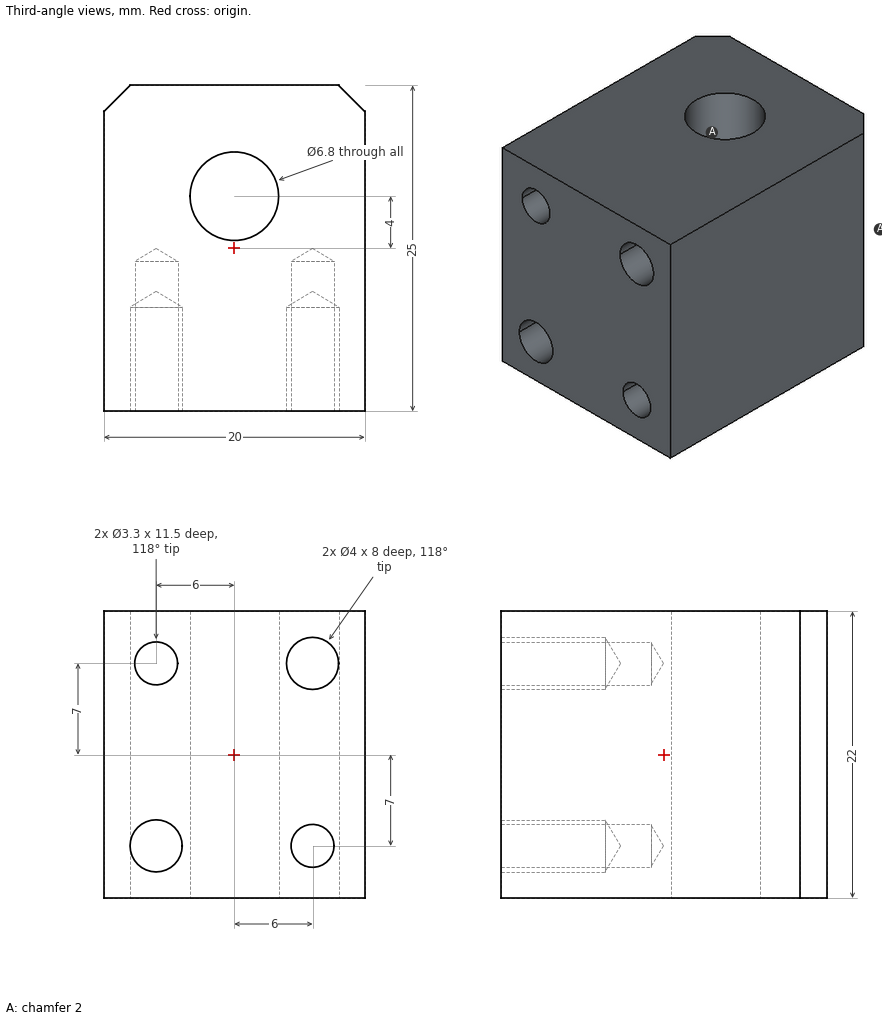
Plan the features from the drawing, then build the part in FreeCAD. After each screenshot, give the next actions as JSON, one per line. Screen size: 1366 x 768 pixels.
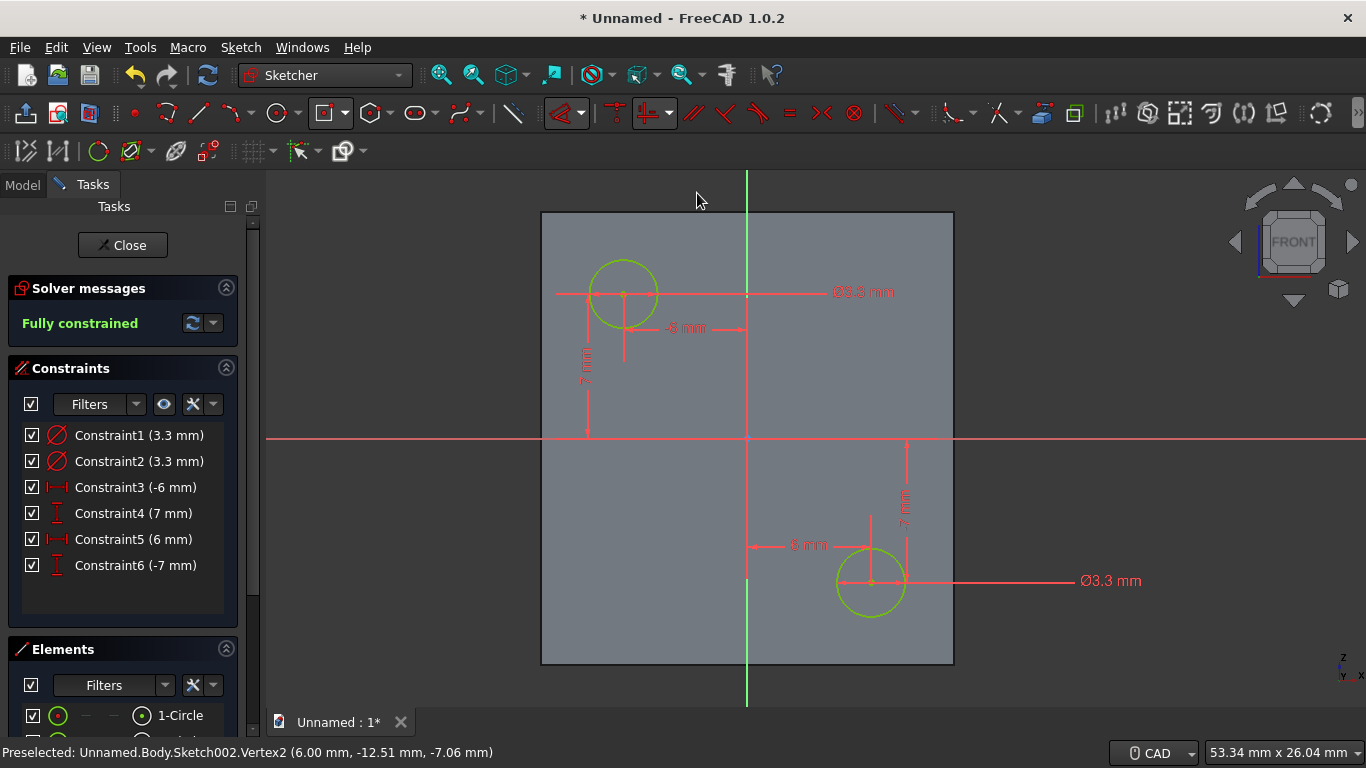
{"action": "left_click", "coordinate": [123, 245]}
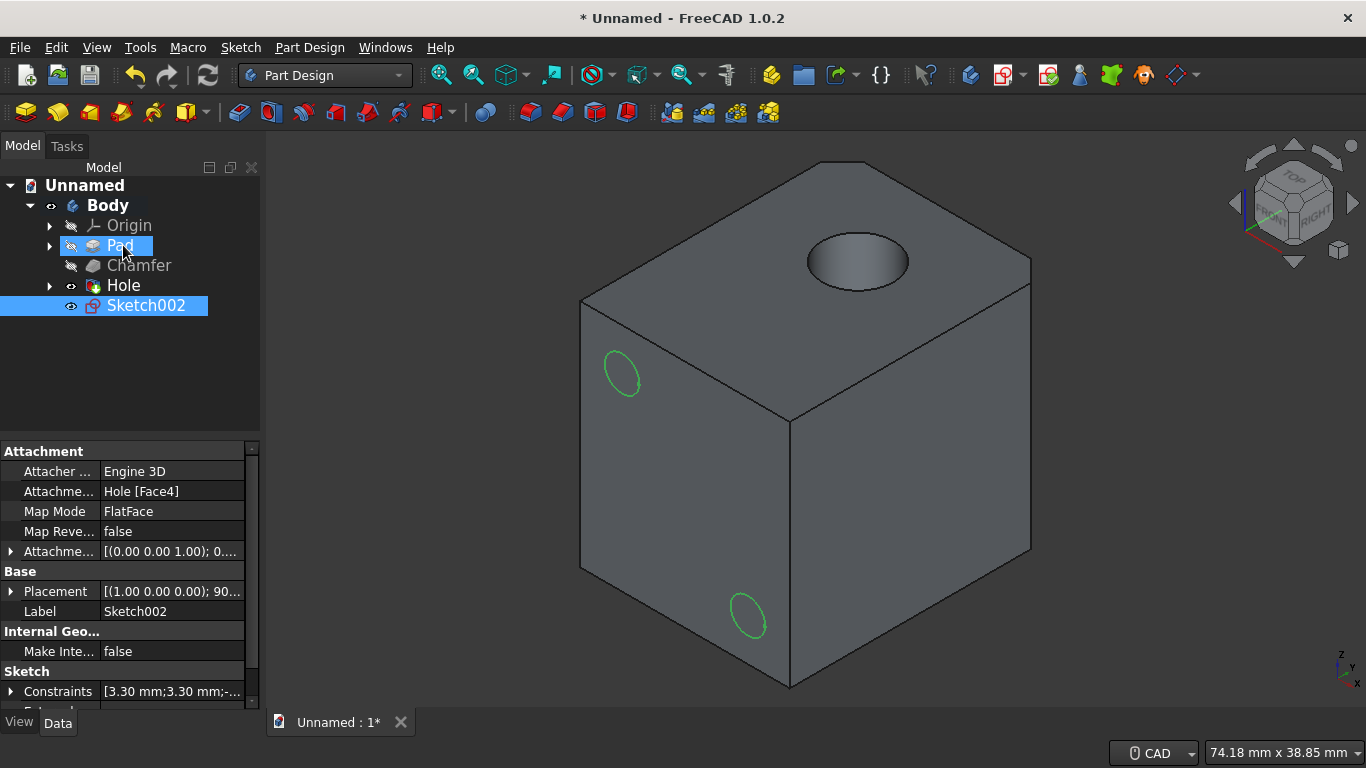
{"action": "left_click", "coordinate": [272, 112]}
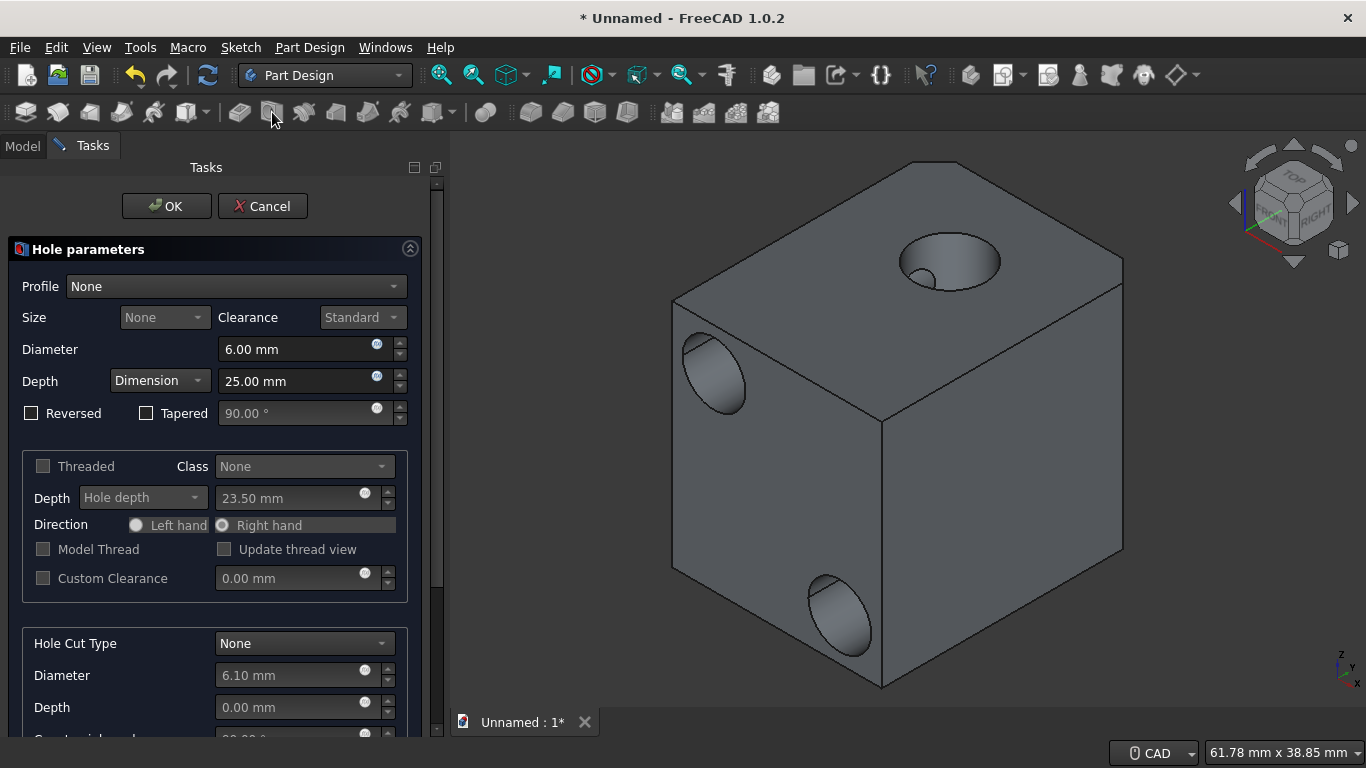
{"action": "triple_click", "coordinate": [305, 349]}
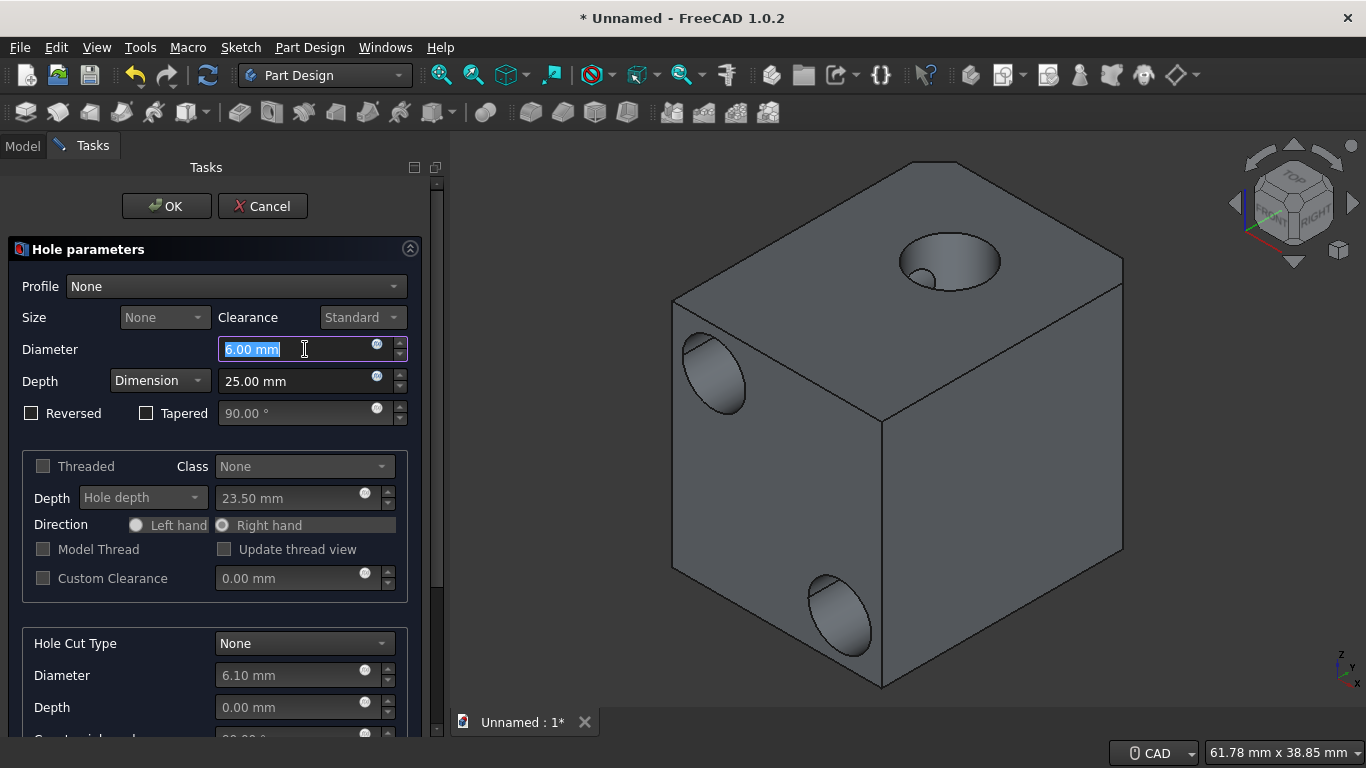
{"action": "type", "text": "3.3"}
{"action": "key", "text": "Tab"}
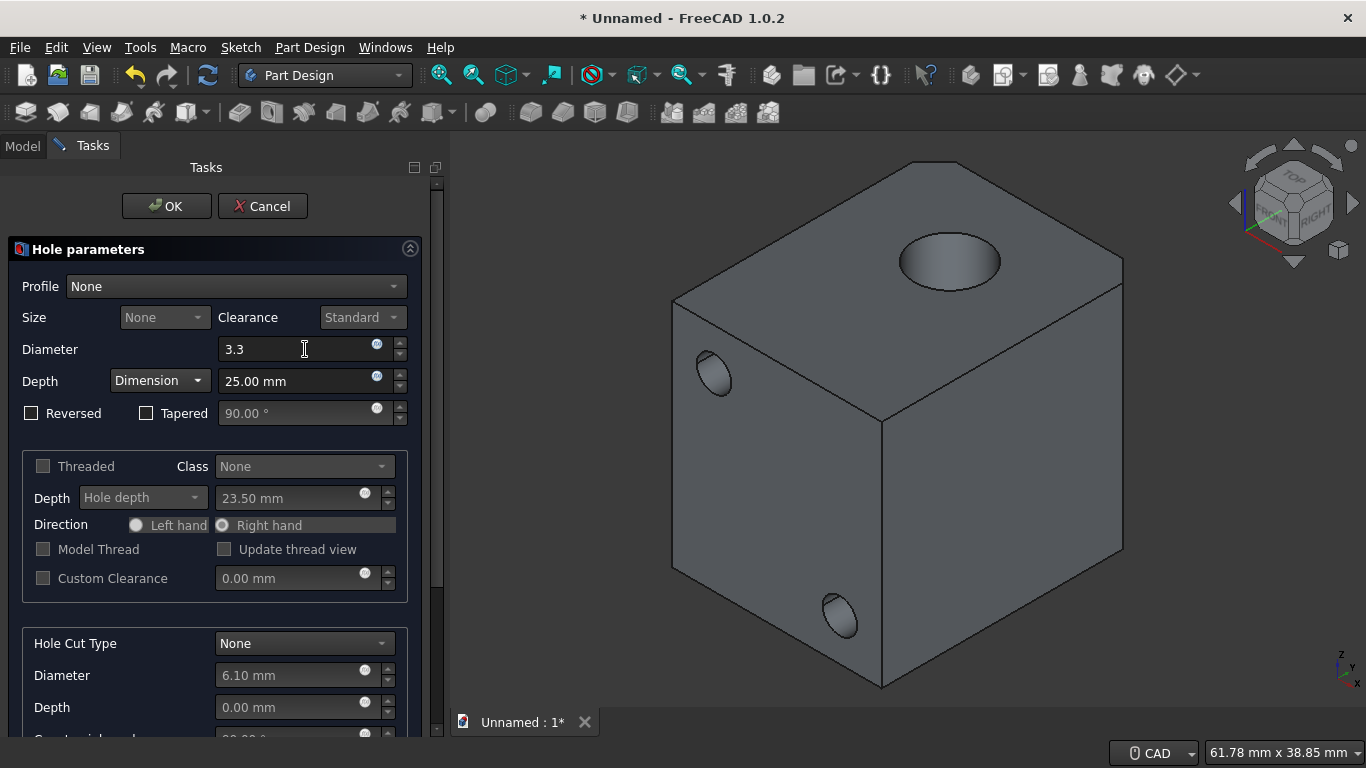
{"action": "triple_click", "coordinate": [305, 381]}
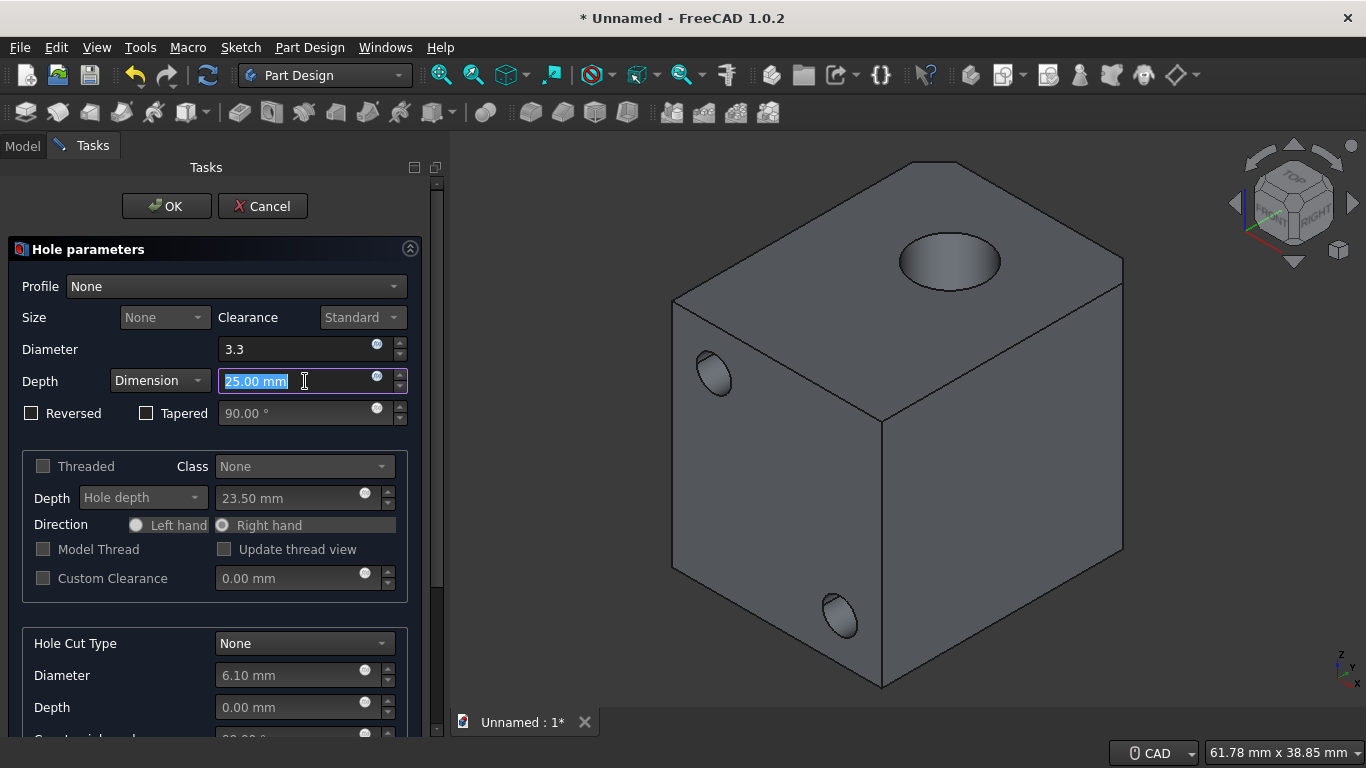
{"action": "type", "text": "11.5"}
{"action": "key", "text": "Tab"}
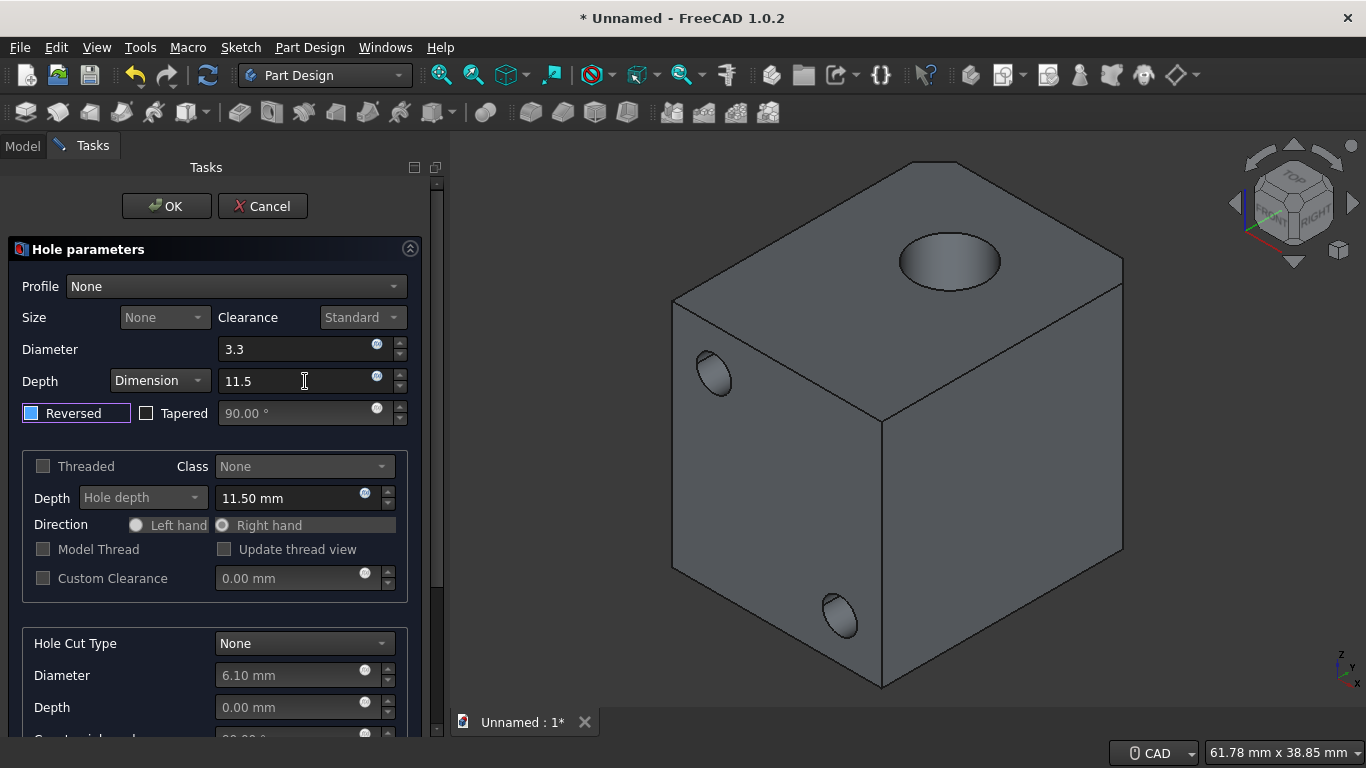
{"action": "left_click", "coordinate": [167, 206]}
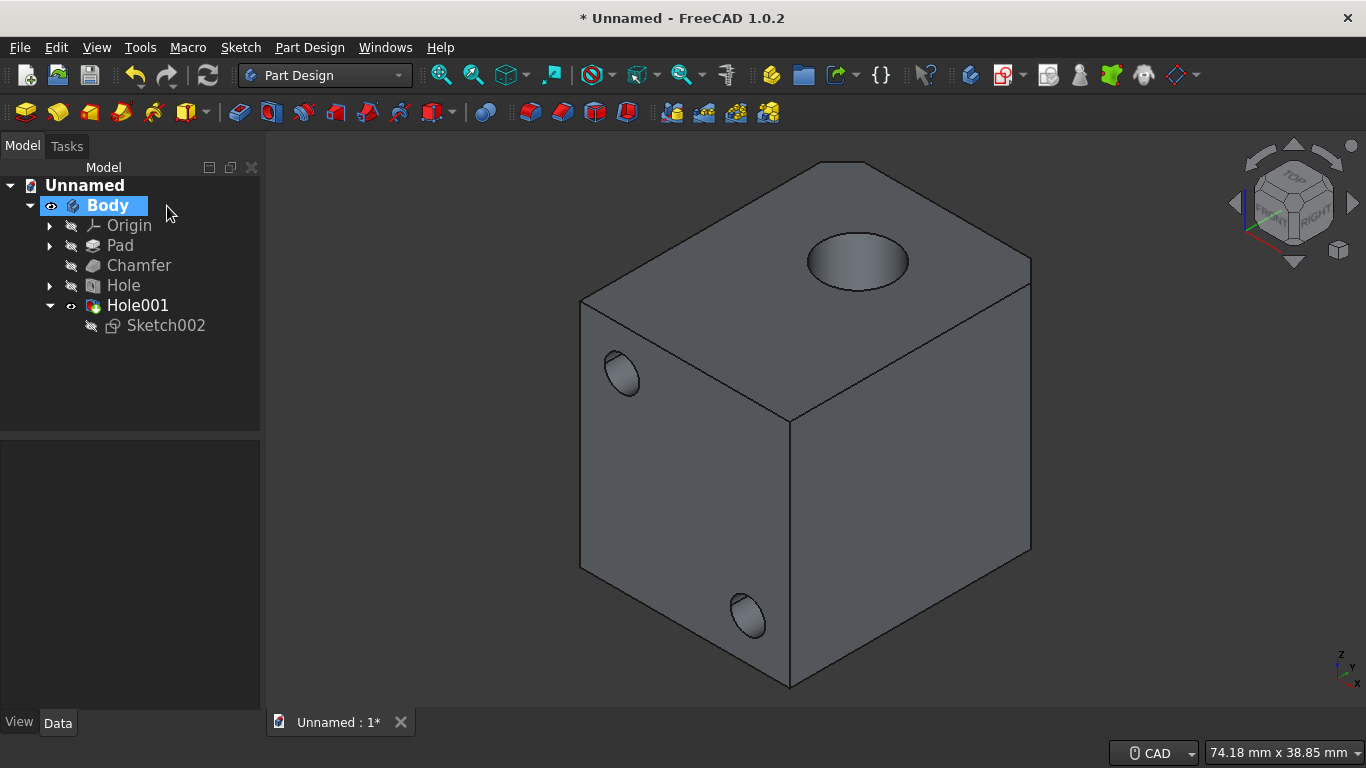
{"action": "left_click", "coordinate": [685, 494]}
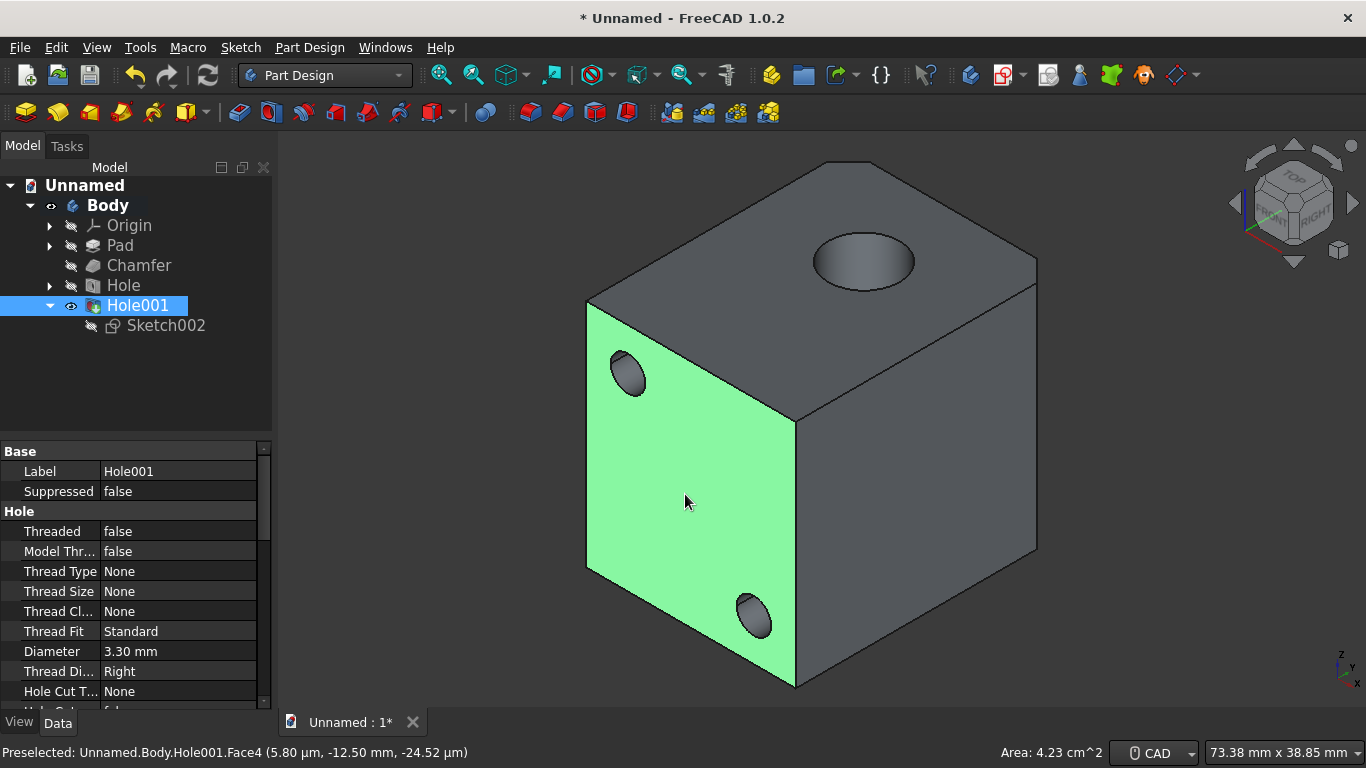
{"action": "left_click", "coordinate": [1004, 76]}